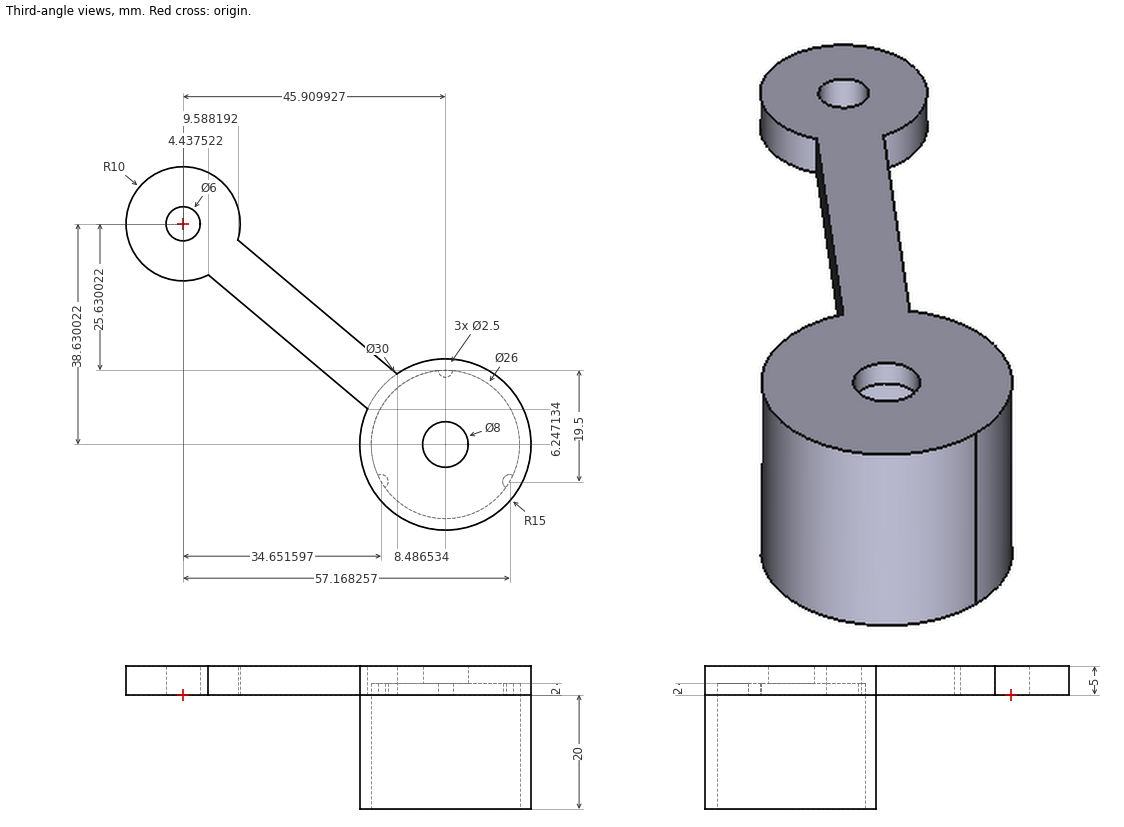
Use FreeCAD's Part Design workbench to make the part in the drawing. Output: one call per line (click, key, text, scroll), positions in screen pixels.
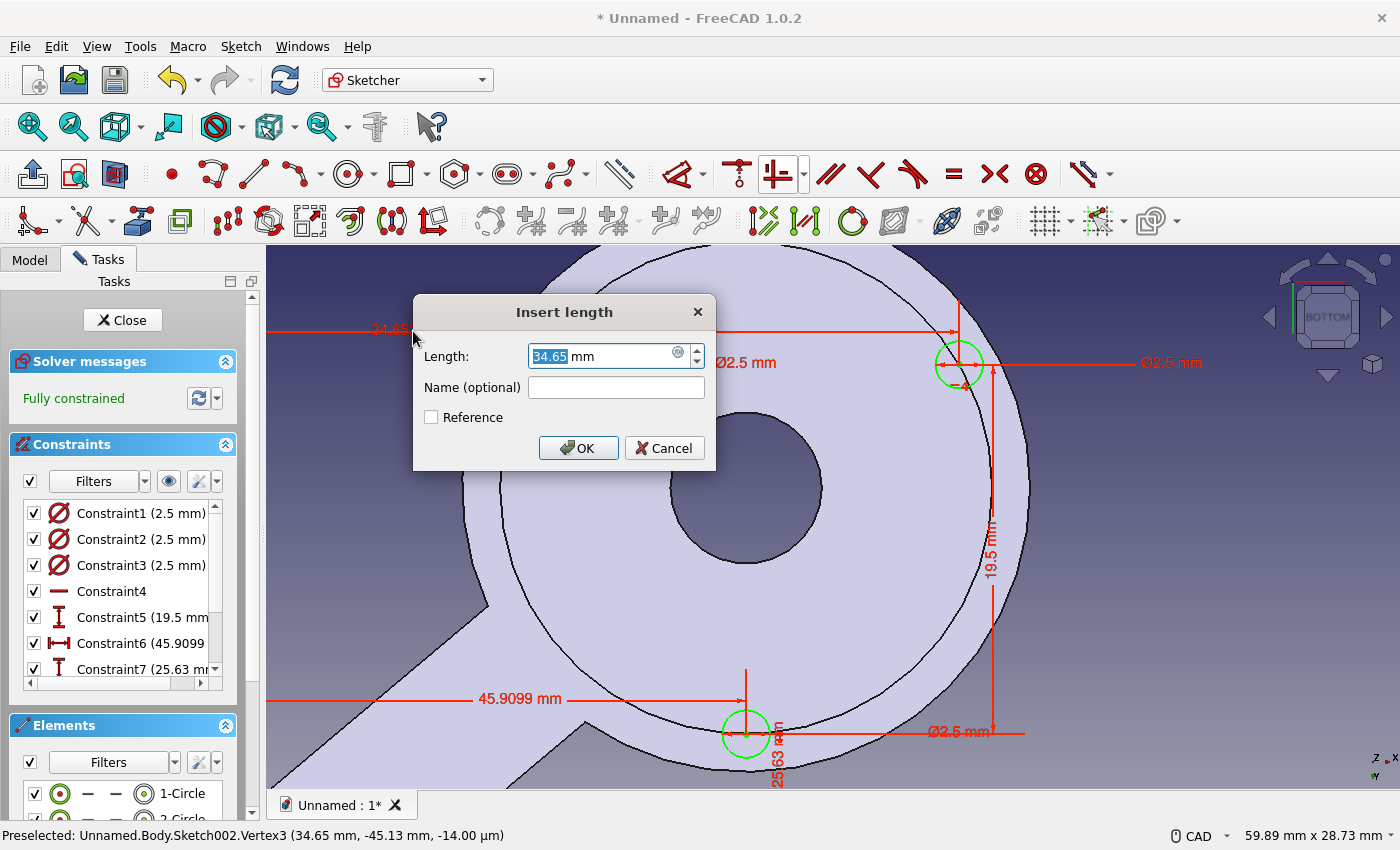
text(34.651597)
key(Return)
key(Escape)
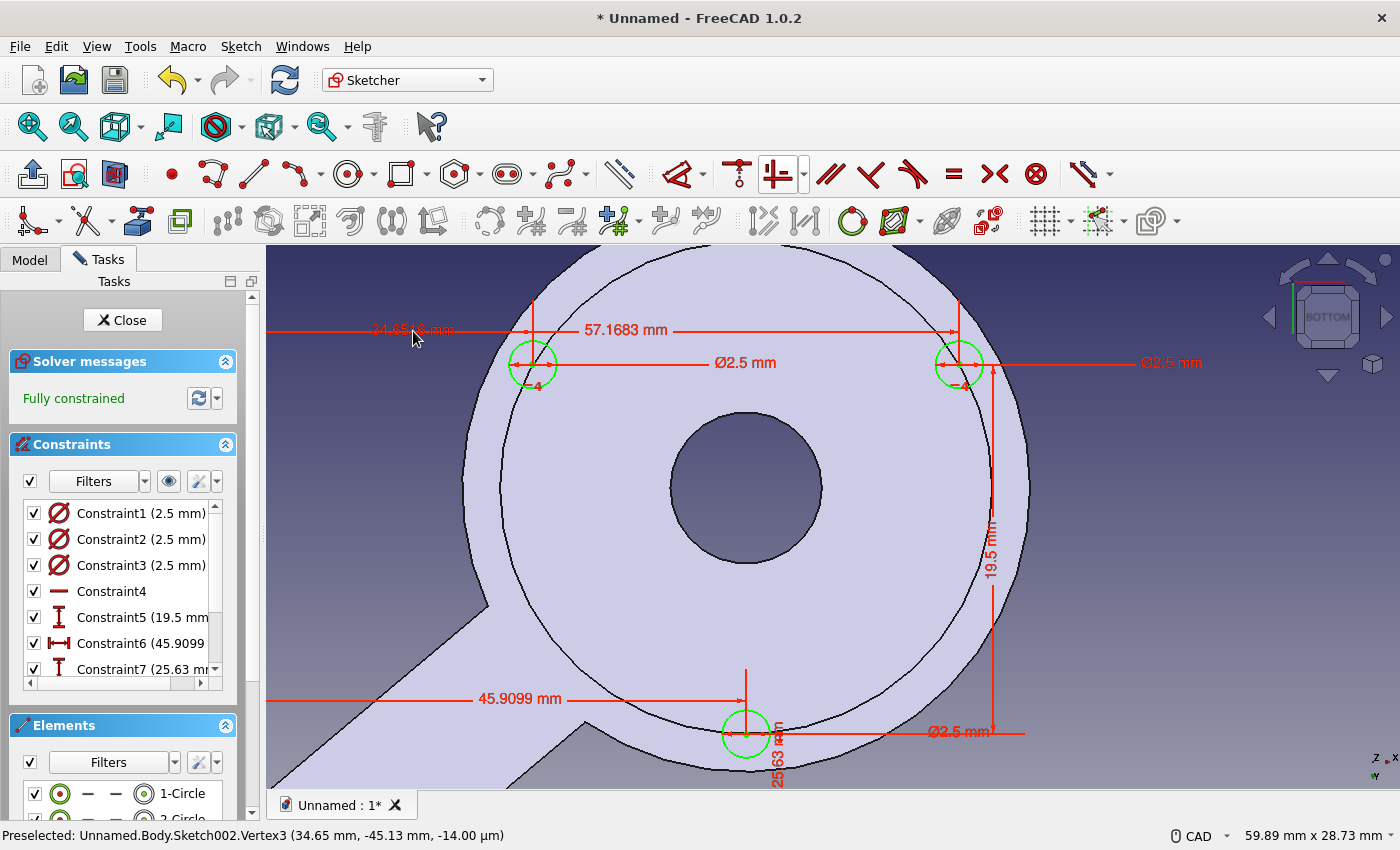
click(123, 320)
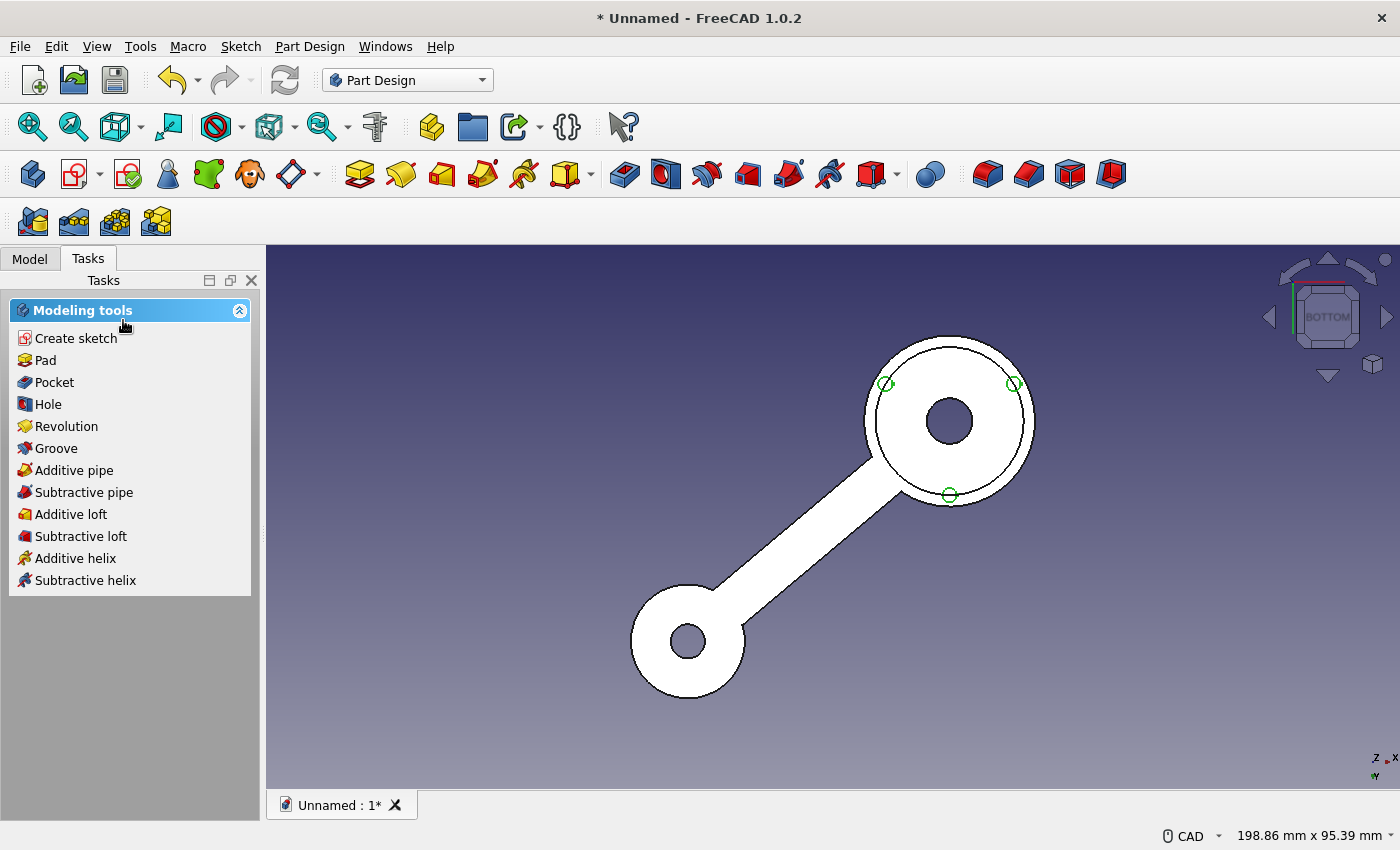
click(360, 174)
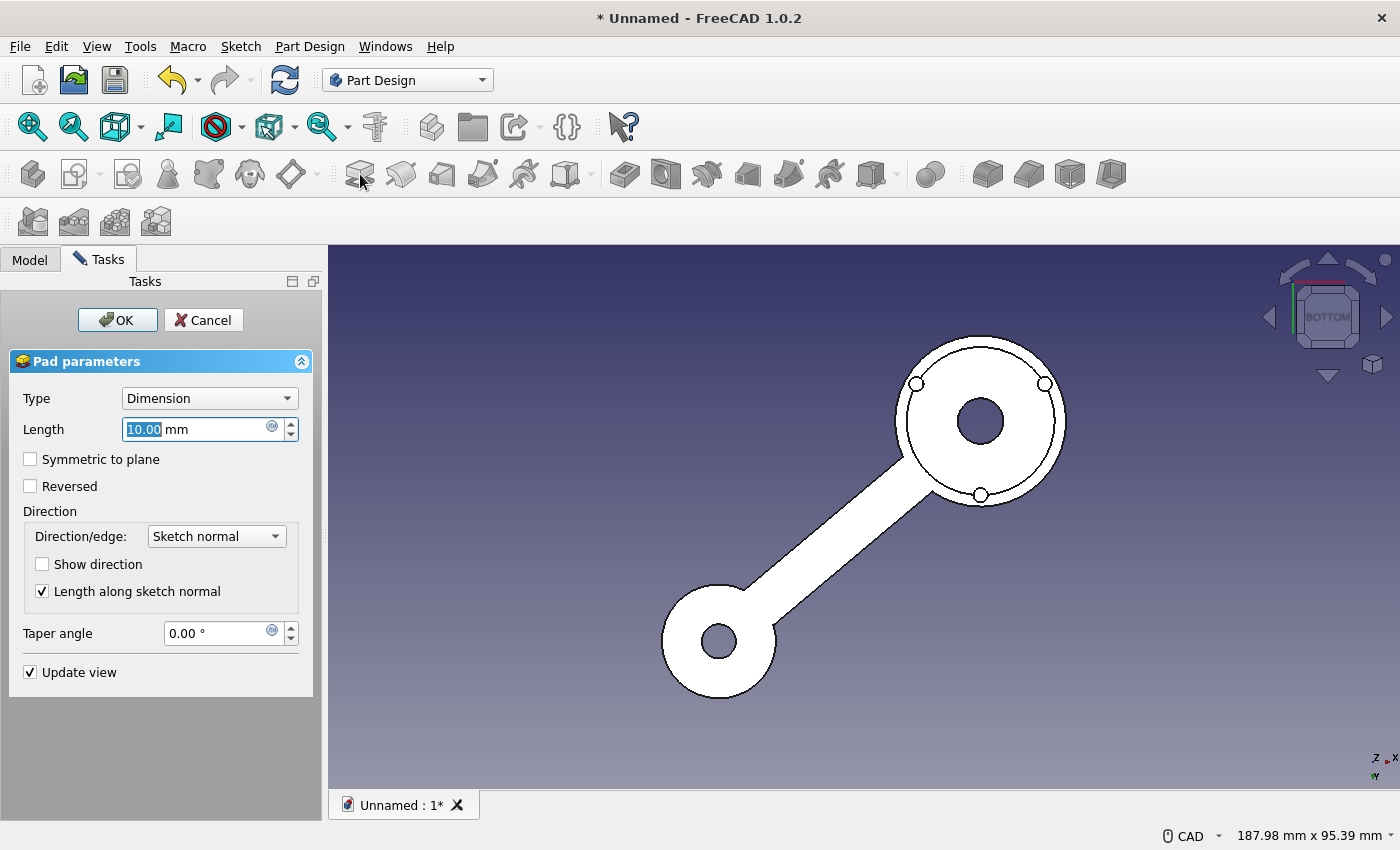
text(2)
key(Tab)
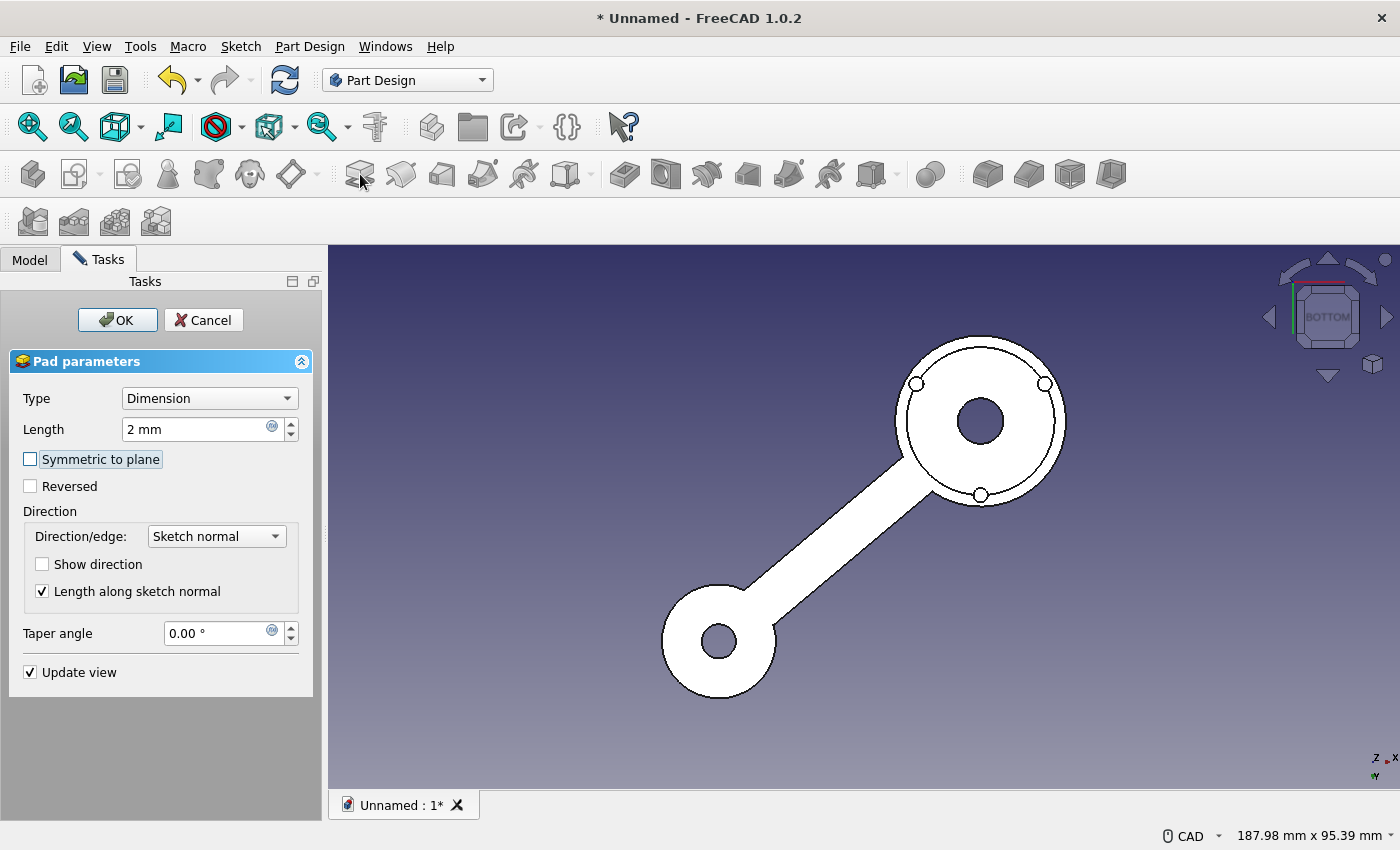
click(31, 486)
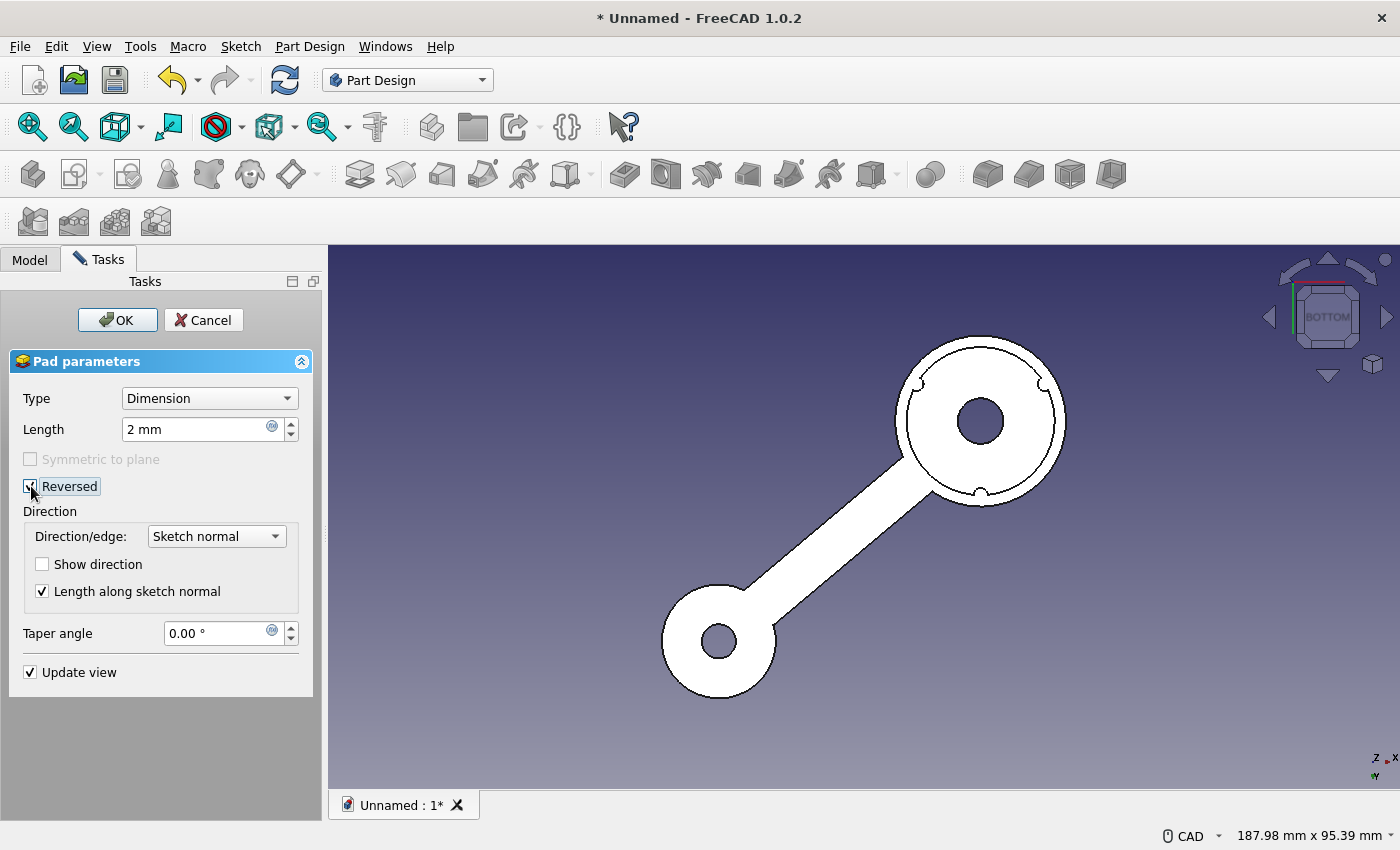
click(118, 320)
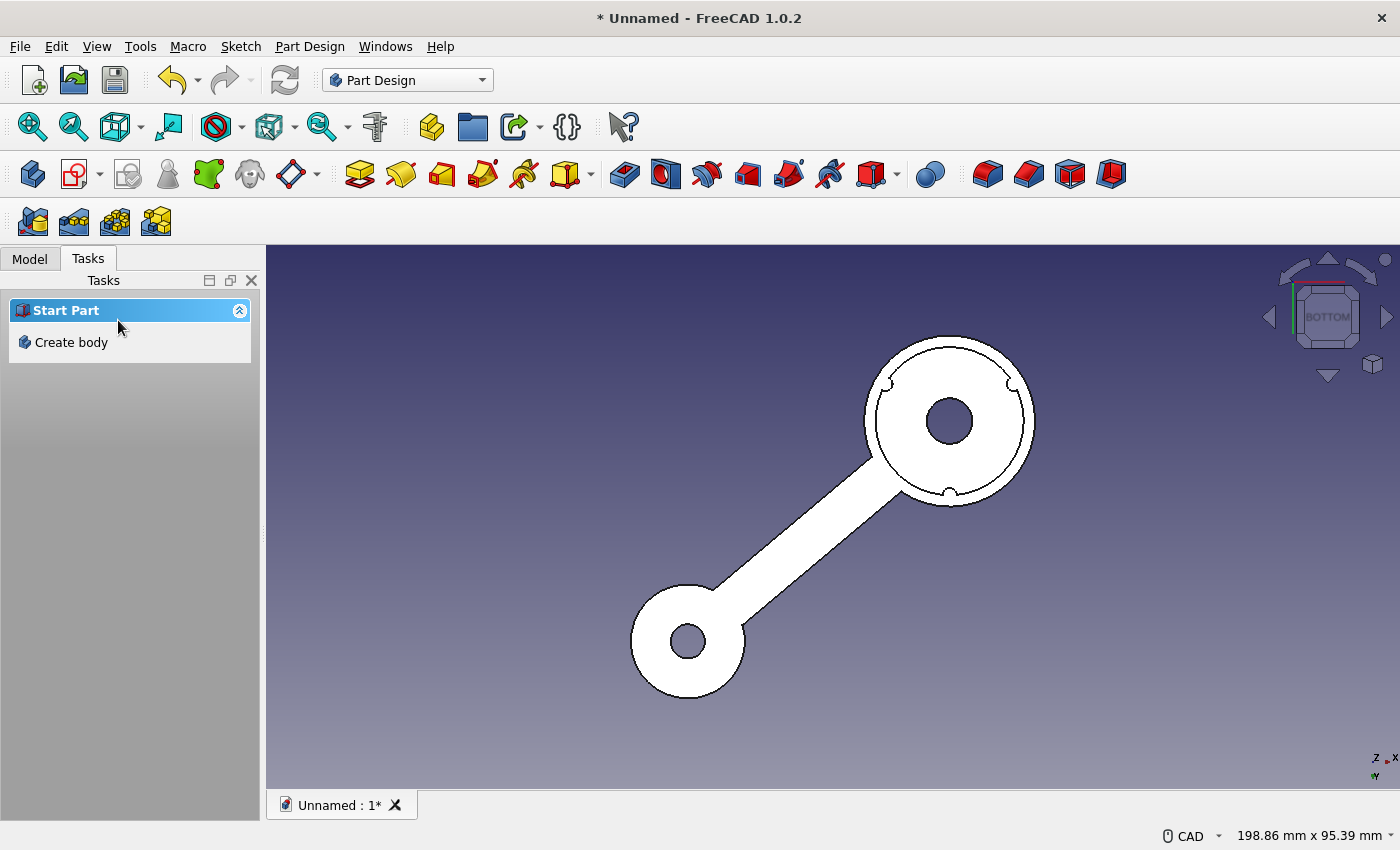
click(30, 258)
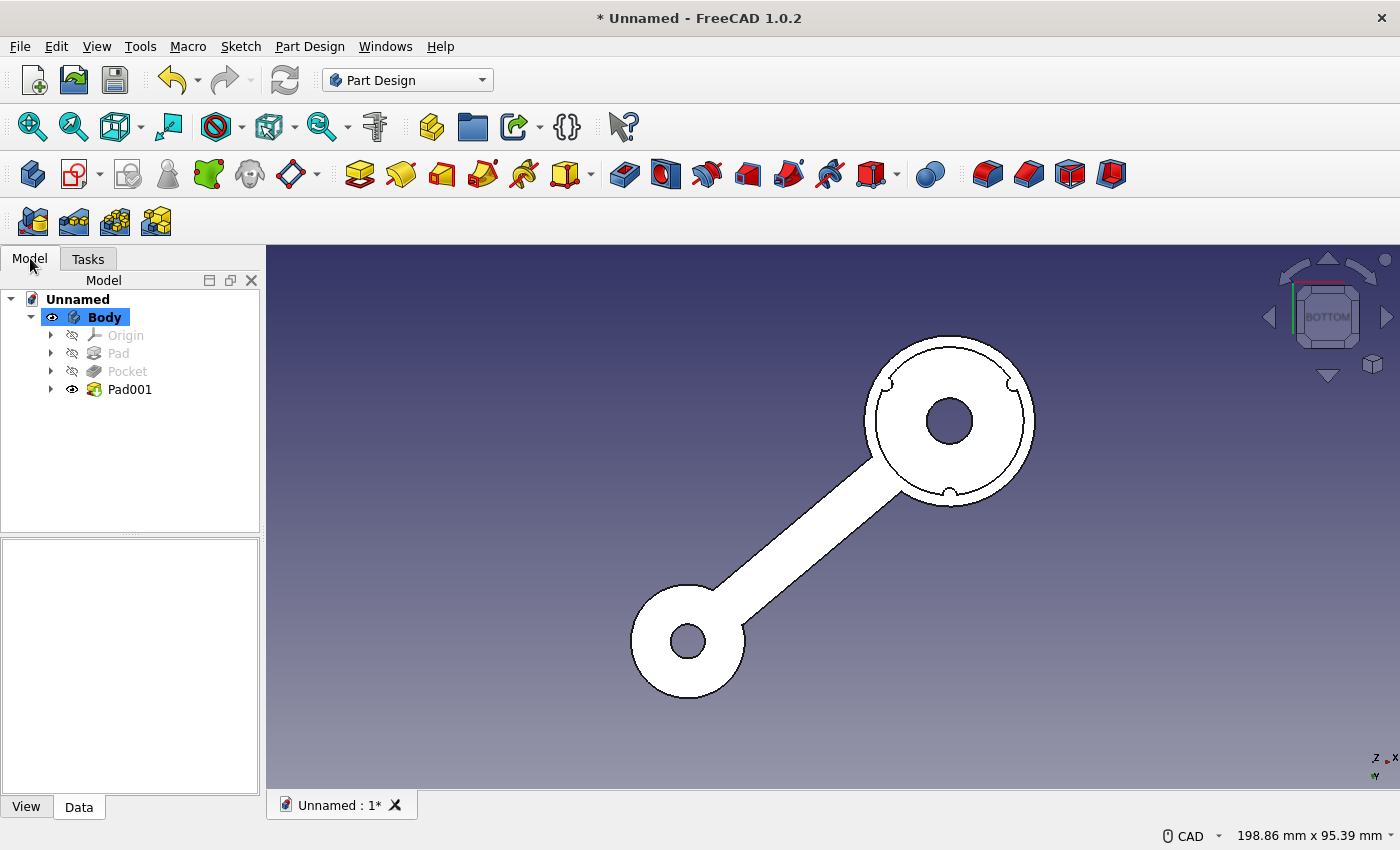
click(51, 335)